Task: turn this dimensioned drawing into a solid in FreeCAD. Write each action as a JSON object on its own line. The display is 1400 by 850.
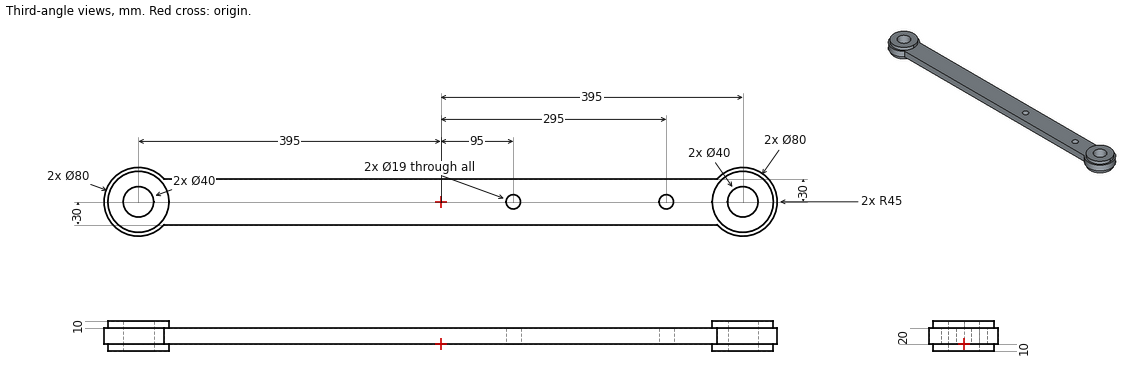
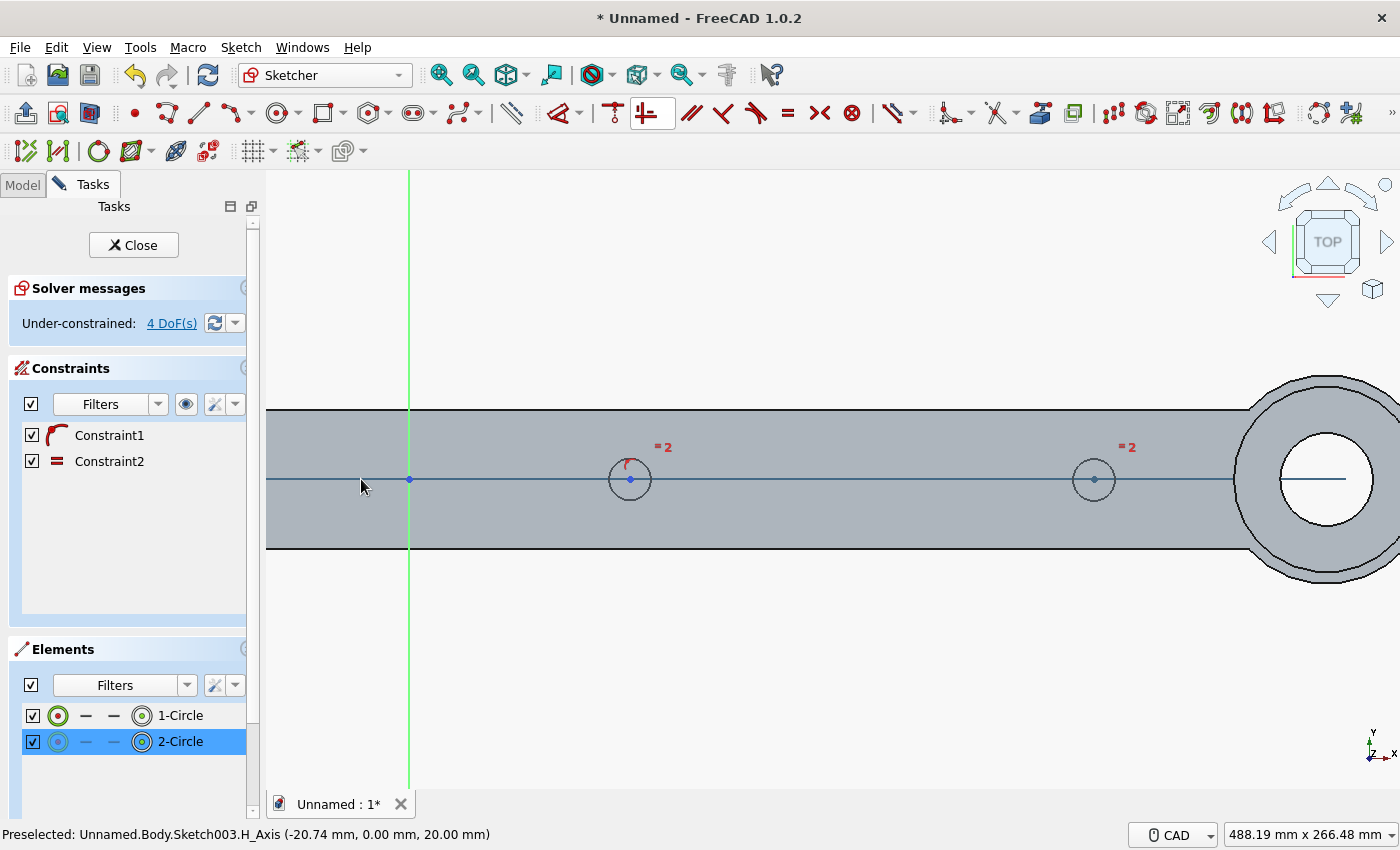
{"action": "key", "text": "c"}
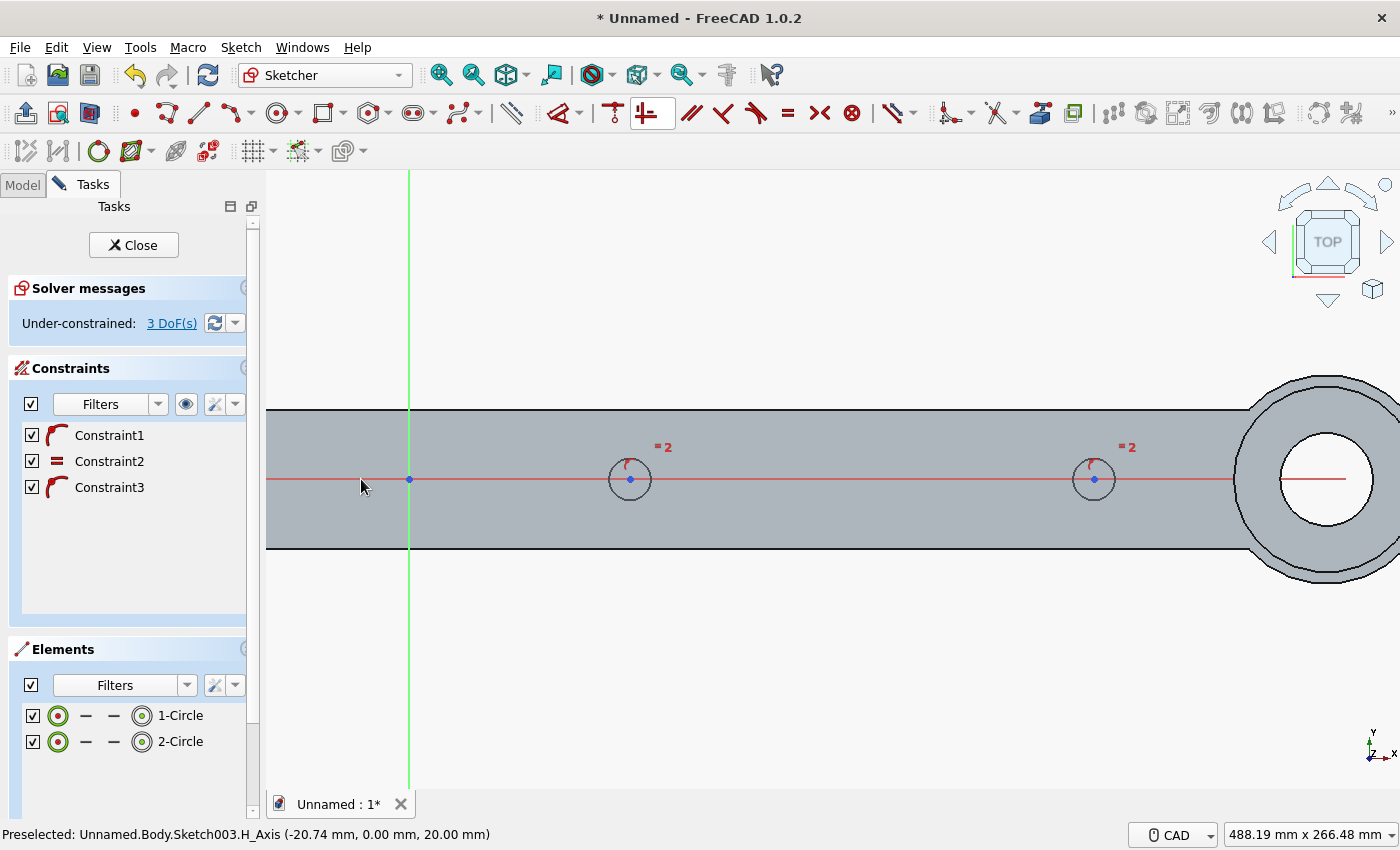
{"action": "left_click", "coordinate": [558, 114]}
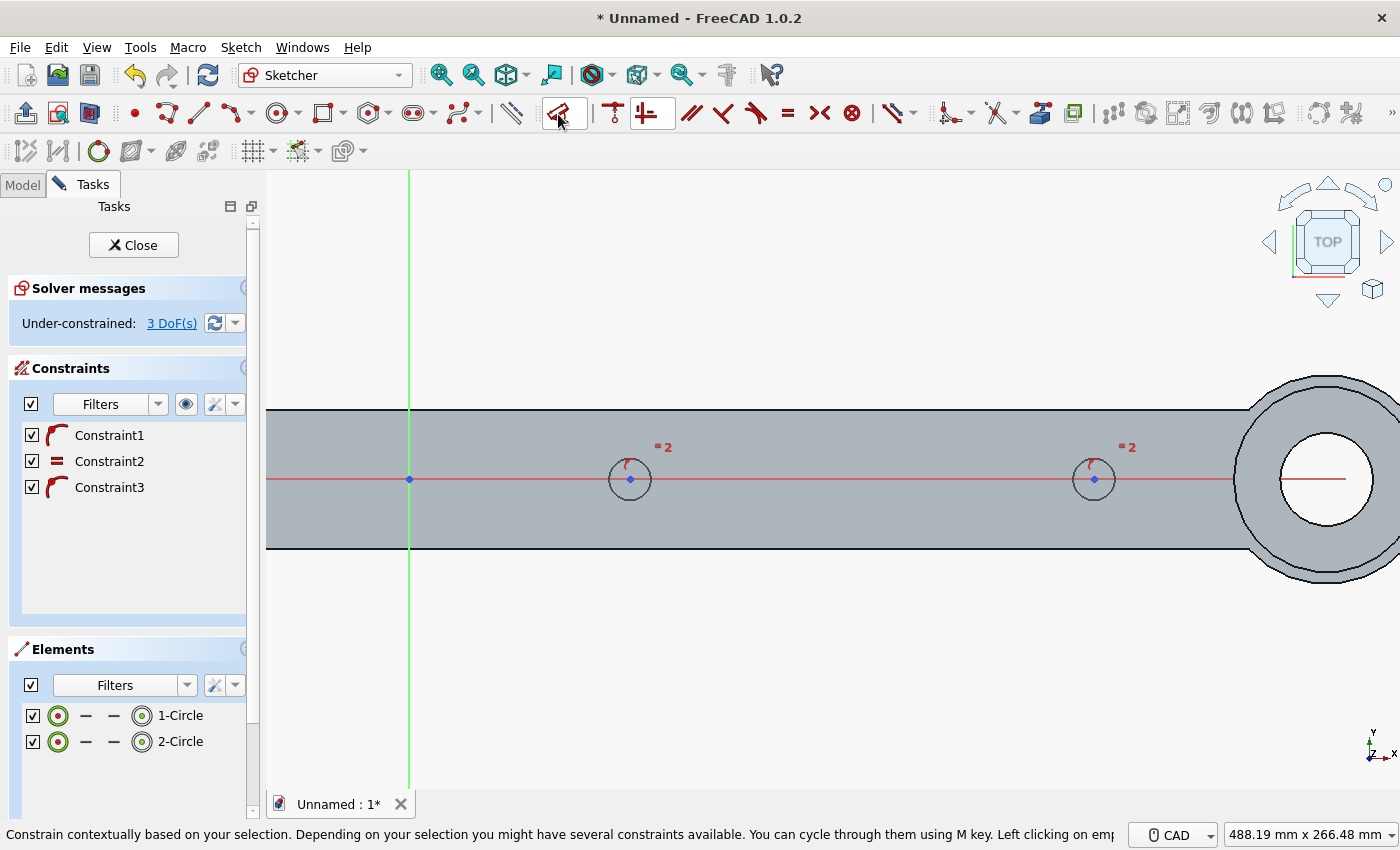
{"action": "left_click", "coordinate": [645, 465]}
{"action": "left_click", "coordinate": [668, 443]}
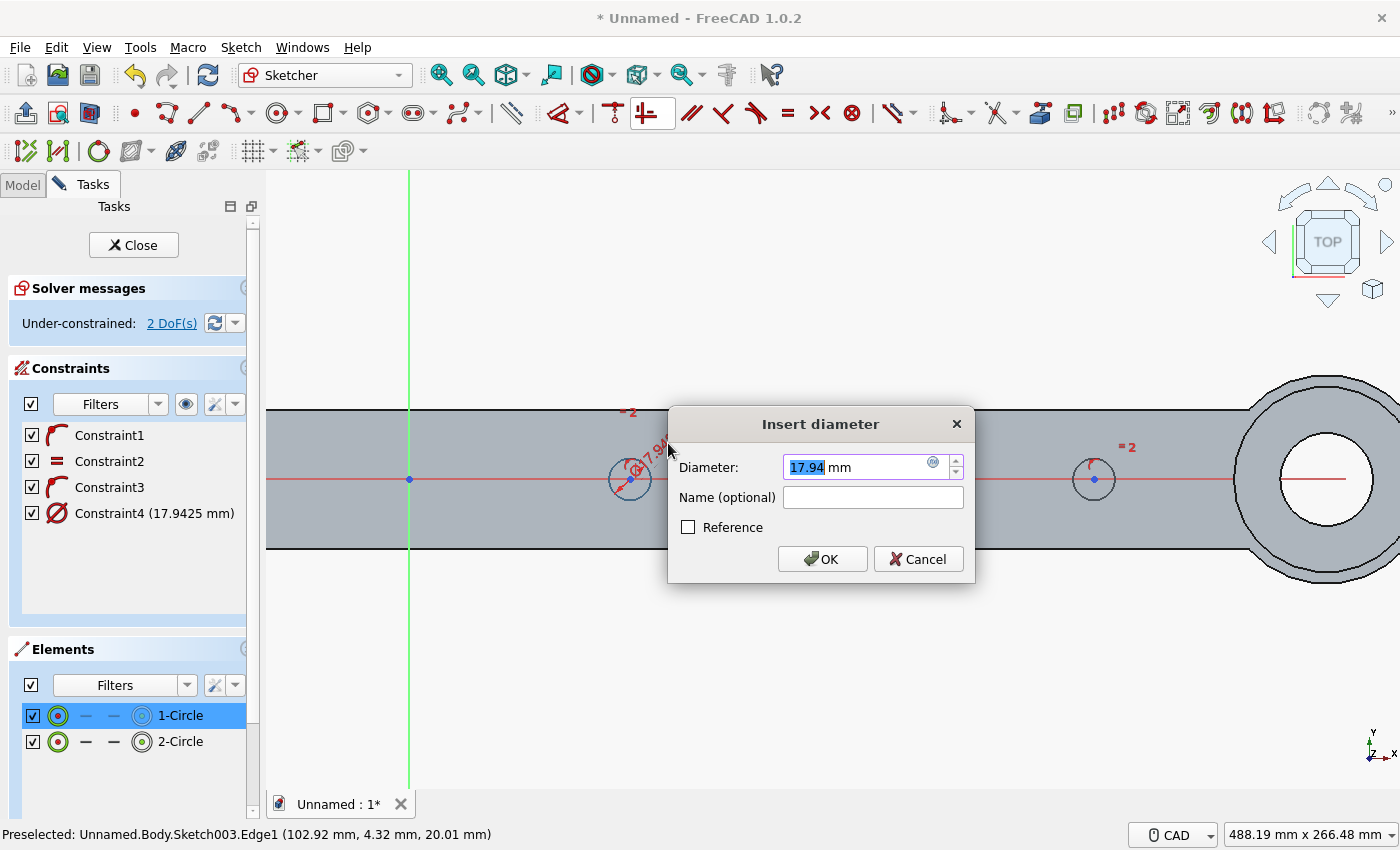
{"action": "type", "text": "19"}
{"action": "key", "text": "Return"}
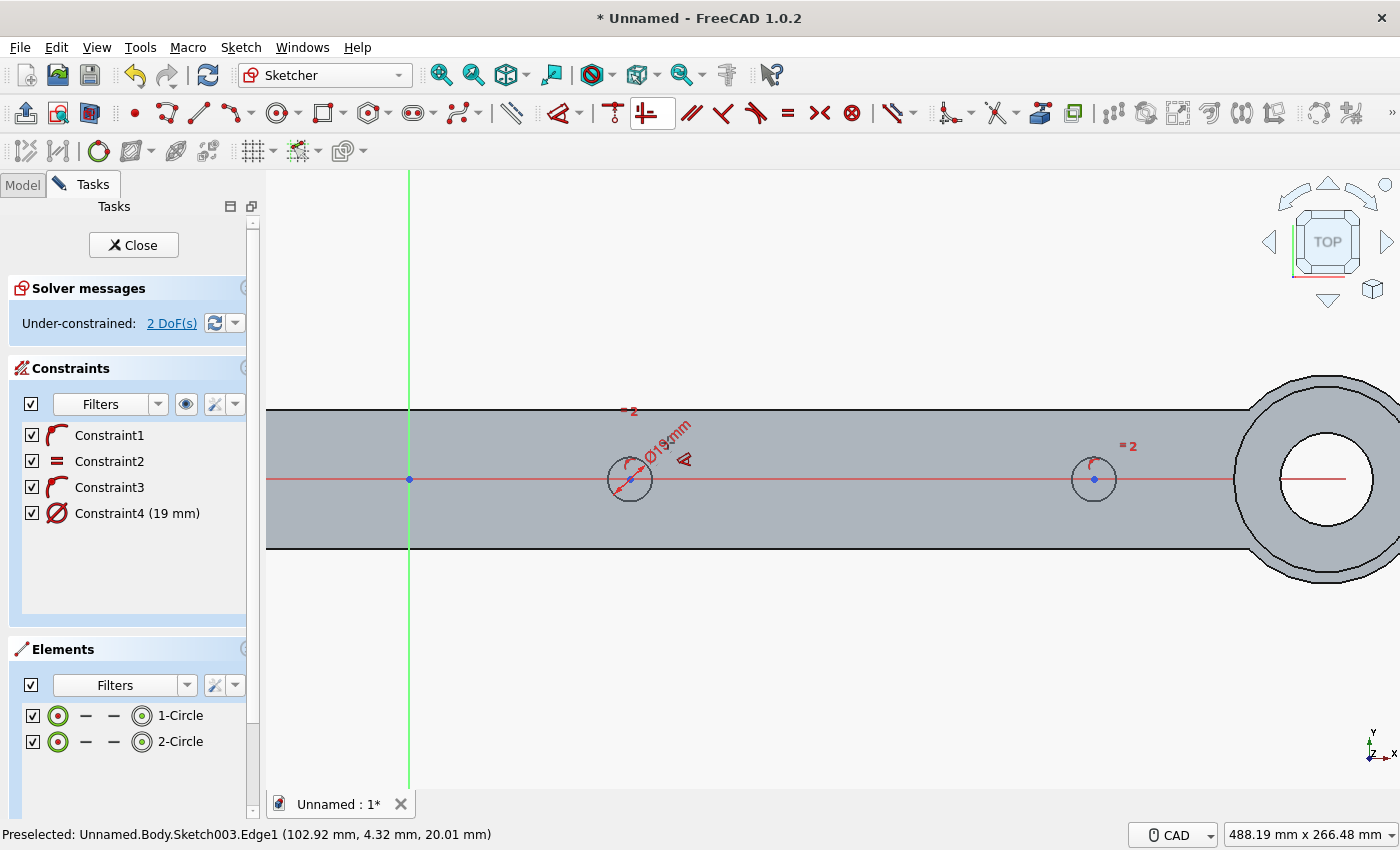
{"action": "left_click", "coordinate": [630, 479]}
{"action": "left_click", "coordinate": [520, 513]}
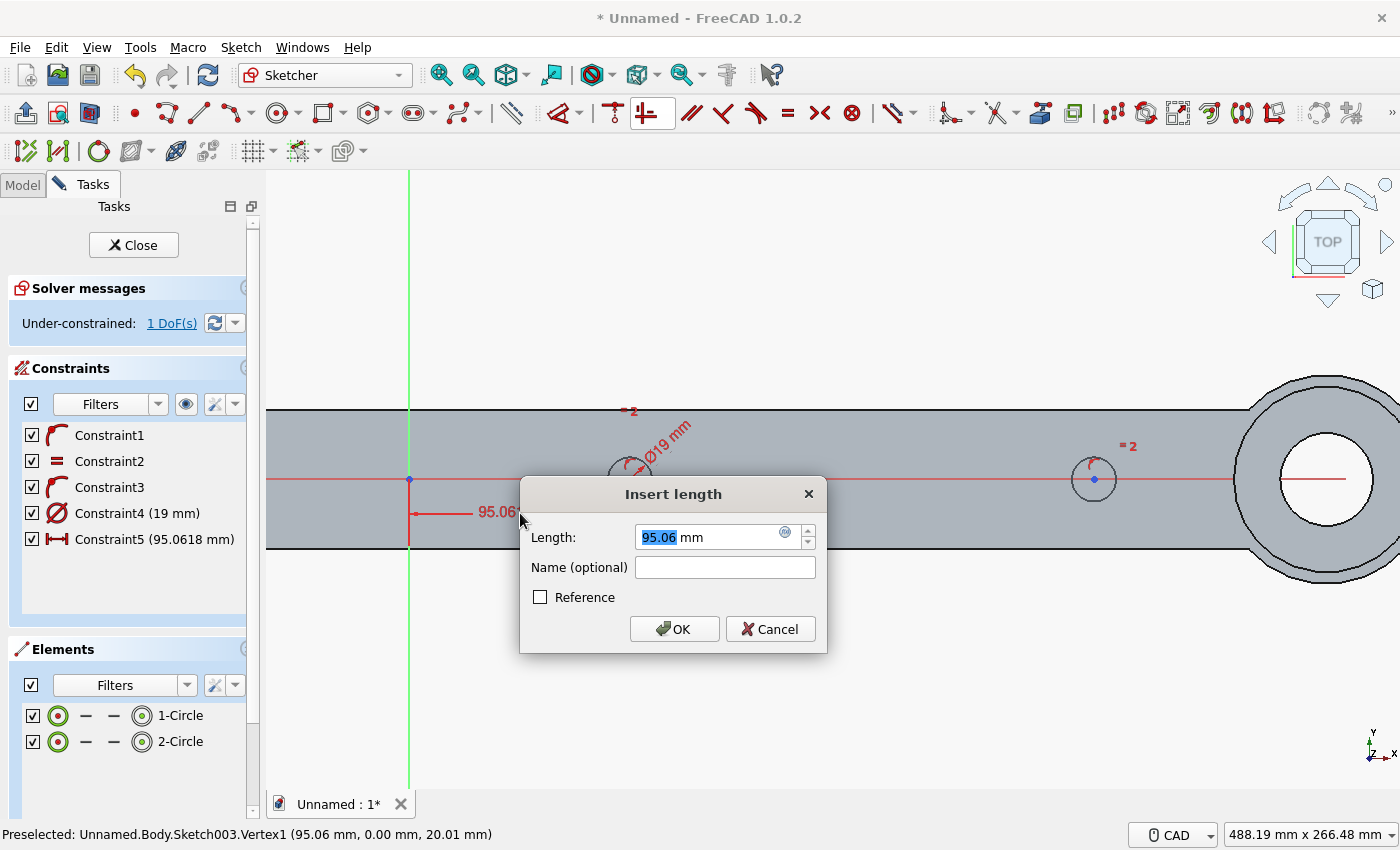
{"action": "type", "text": "95"}
{"action": "key", "text": "Return"}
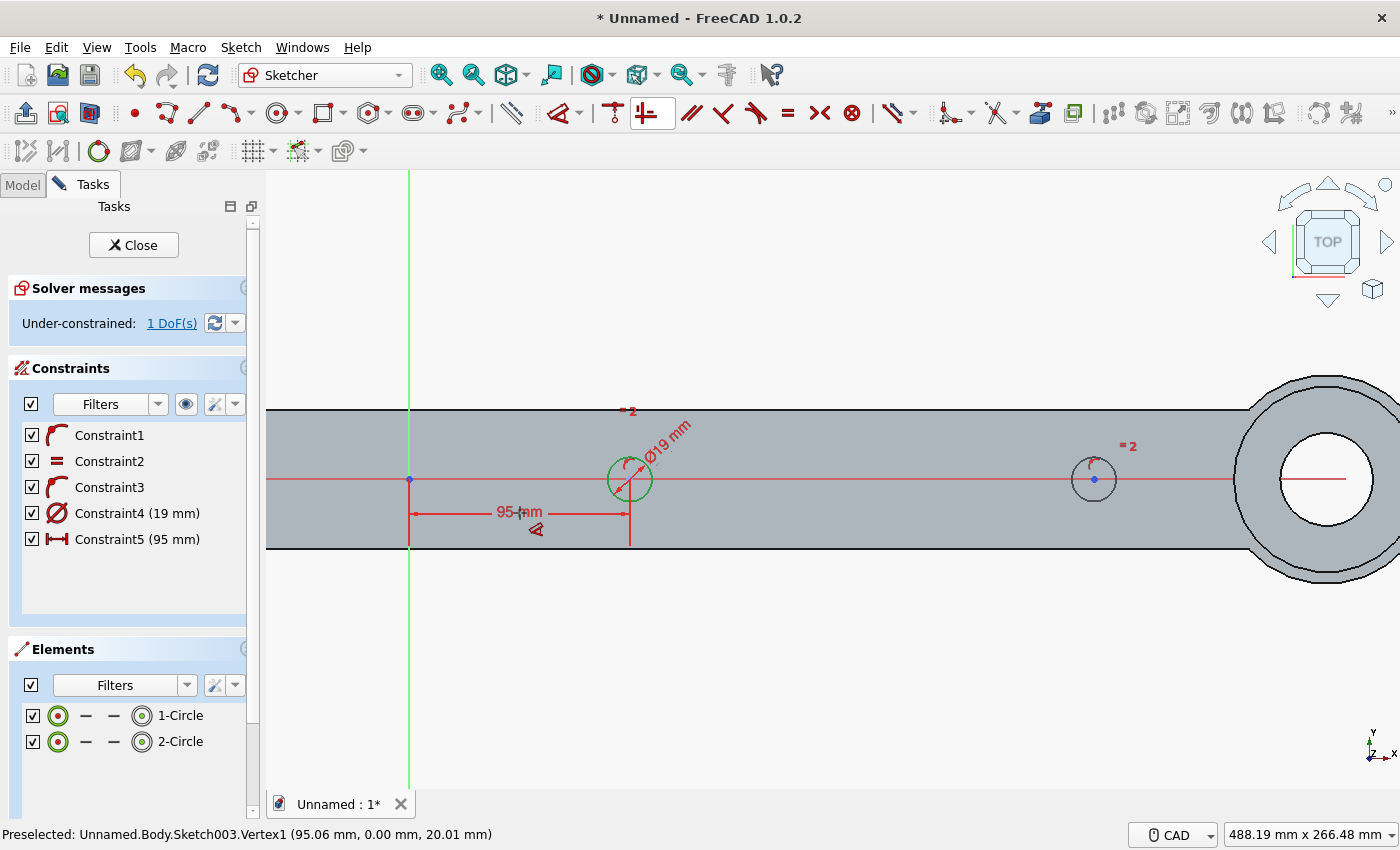
{"action": "left_click", "coordinate": [1094, 479]}
{"action": "left_click", "coordinate": [752, 513]}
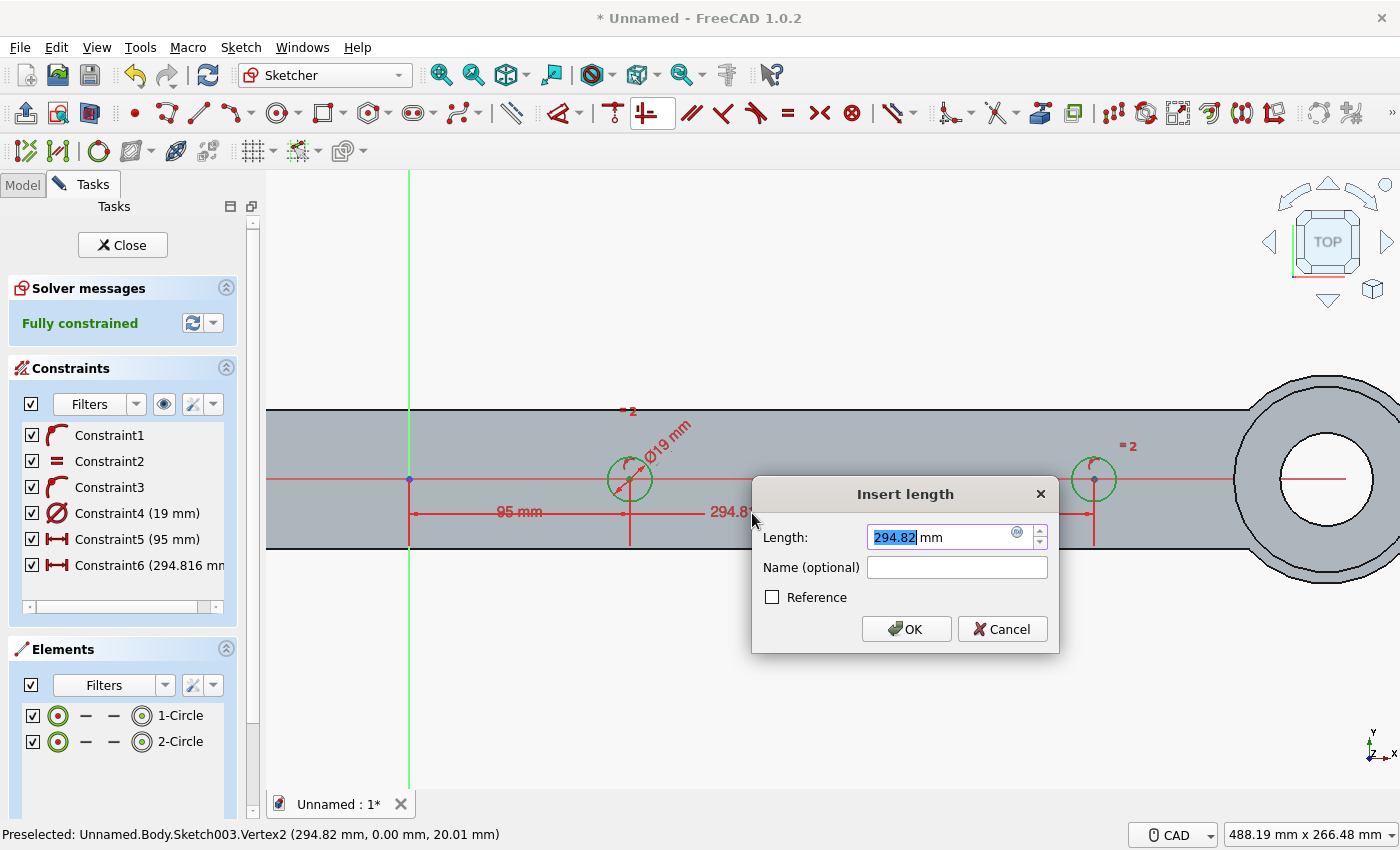
{"action": "type", "text": "295"}
{"action": "key", "text": "Return"}
{"action": "key", "text": "Escape"}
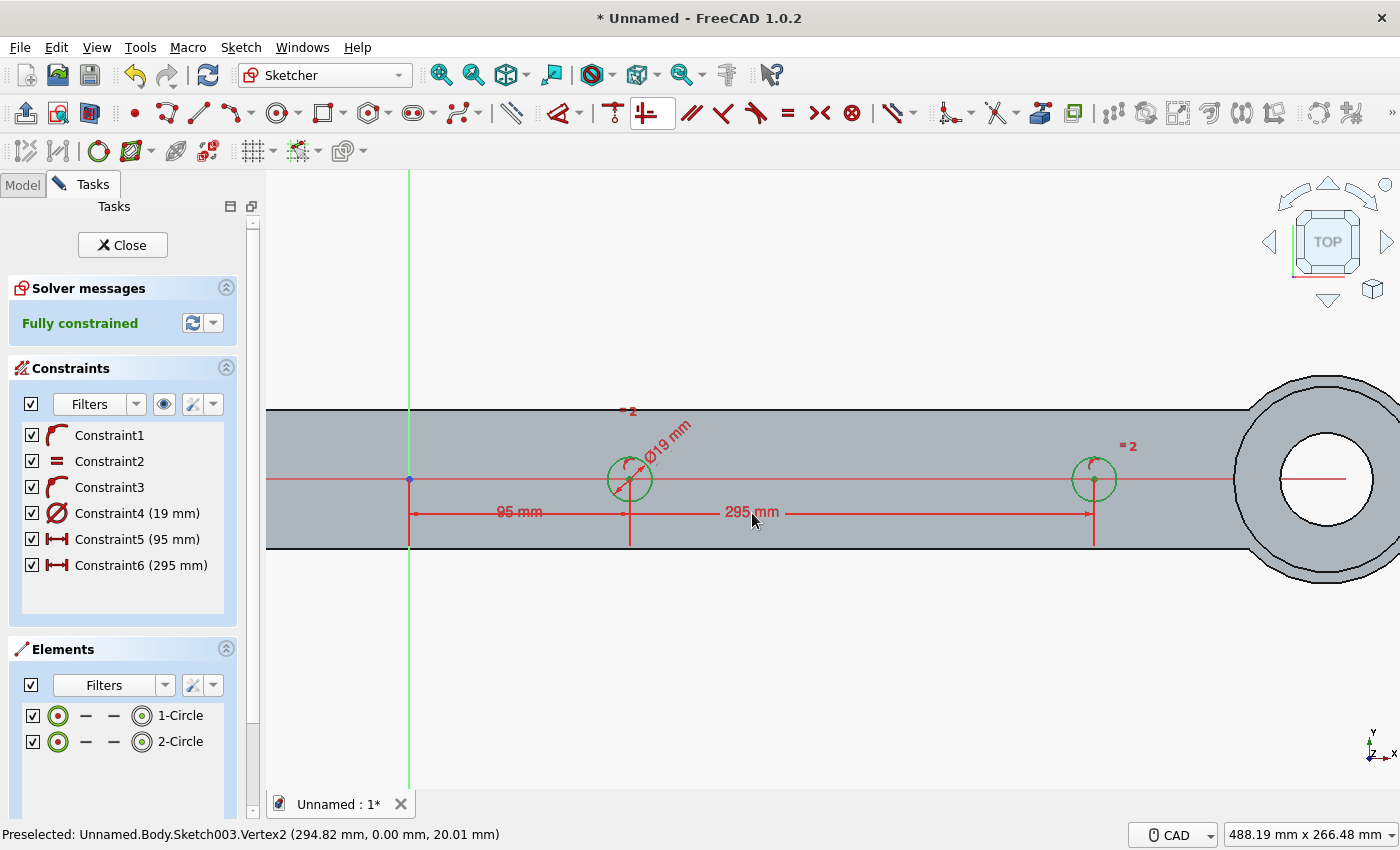
{"action": "left_click", "coordinate": [123, 245]}